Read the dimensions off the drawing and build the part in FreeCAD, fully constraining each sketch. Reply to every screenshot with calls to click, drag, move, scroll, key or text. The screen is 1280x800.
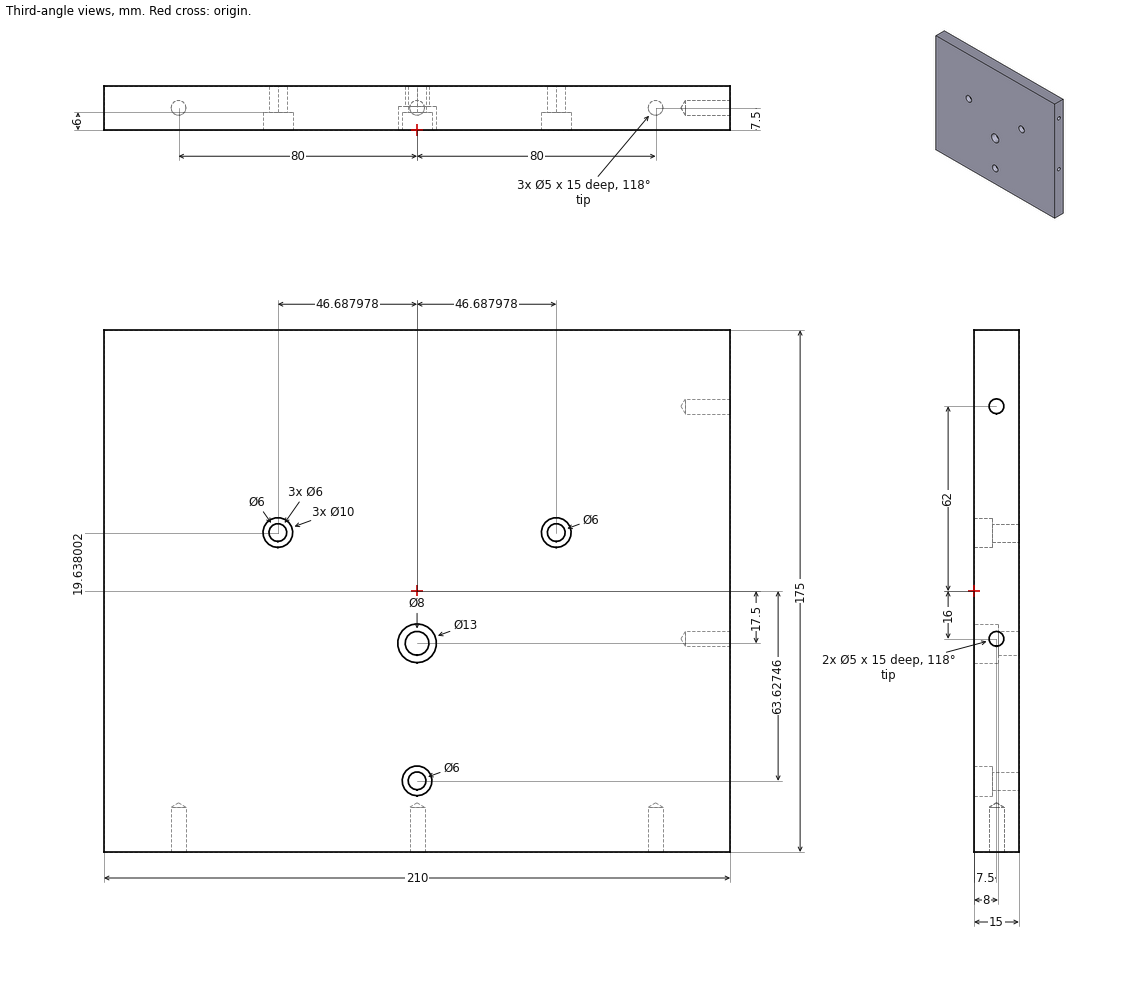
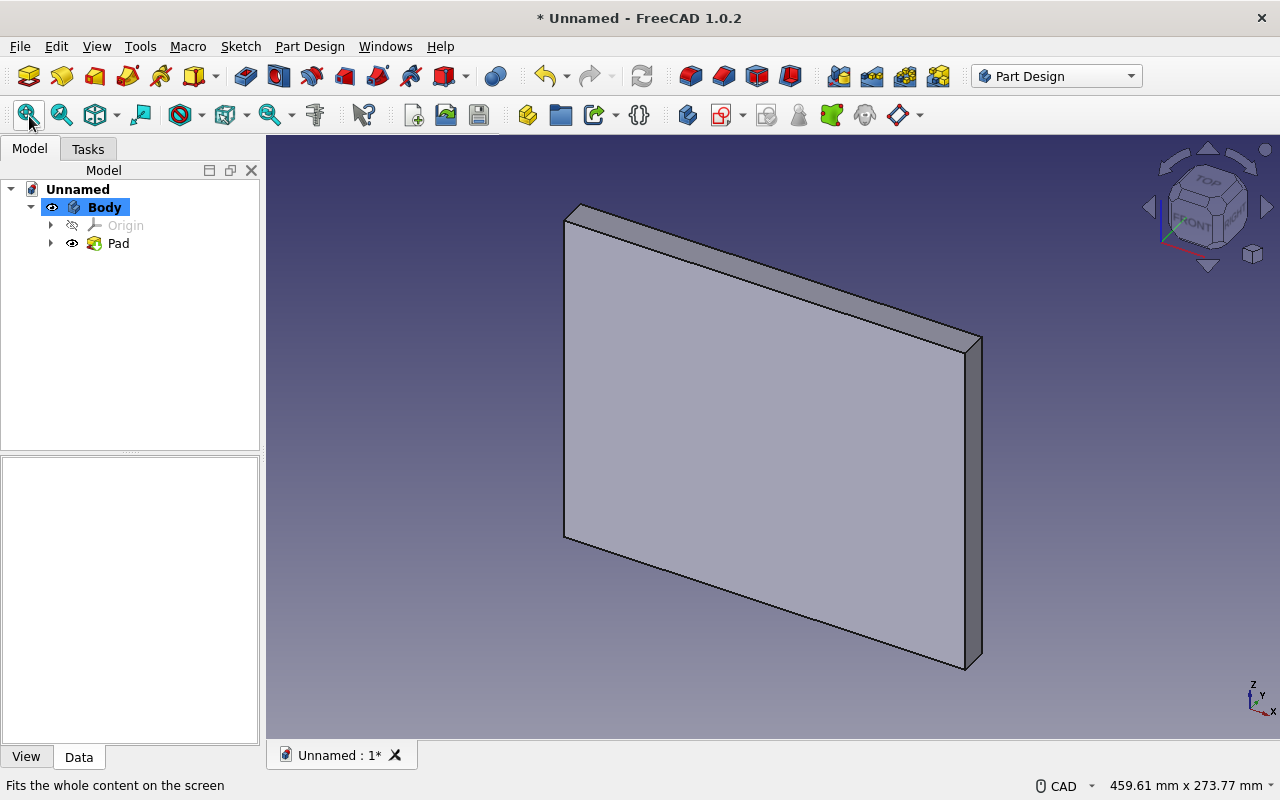
click(720, 116)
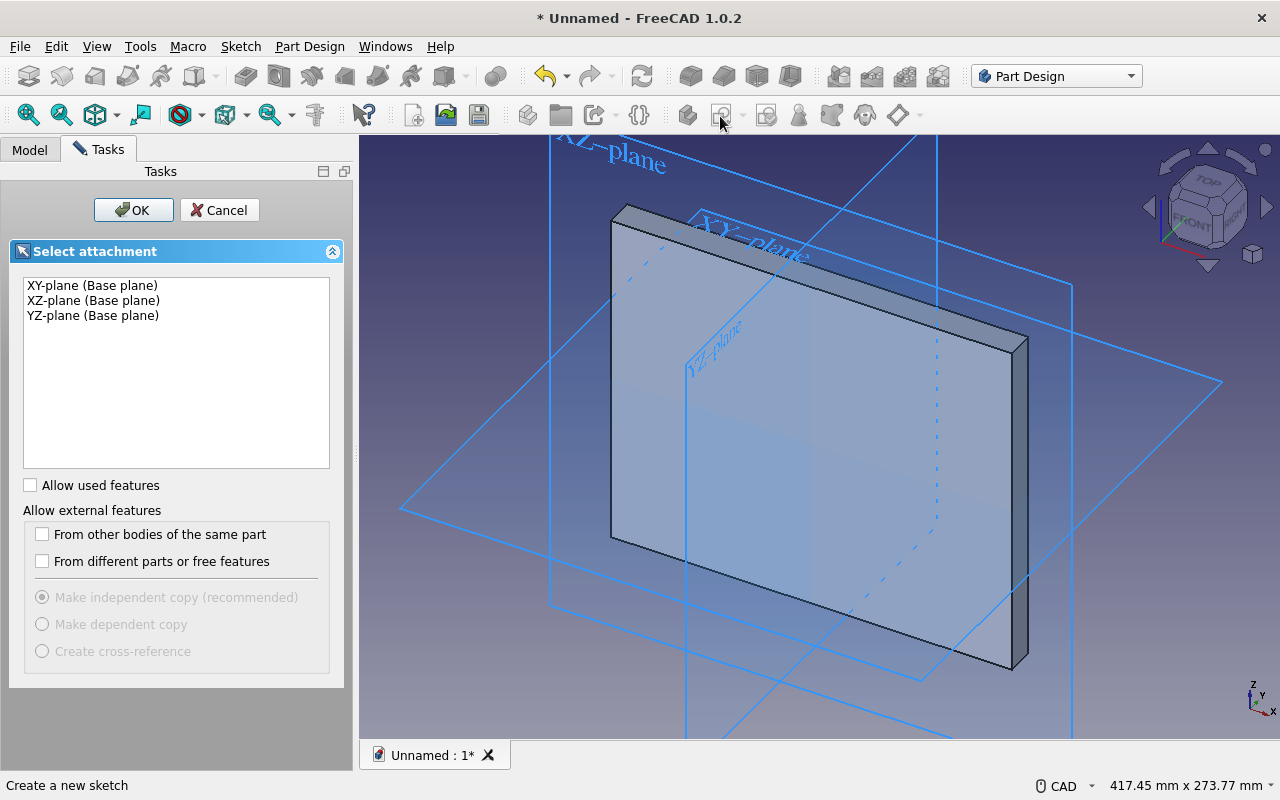
click(84, 300)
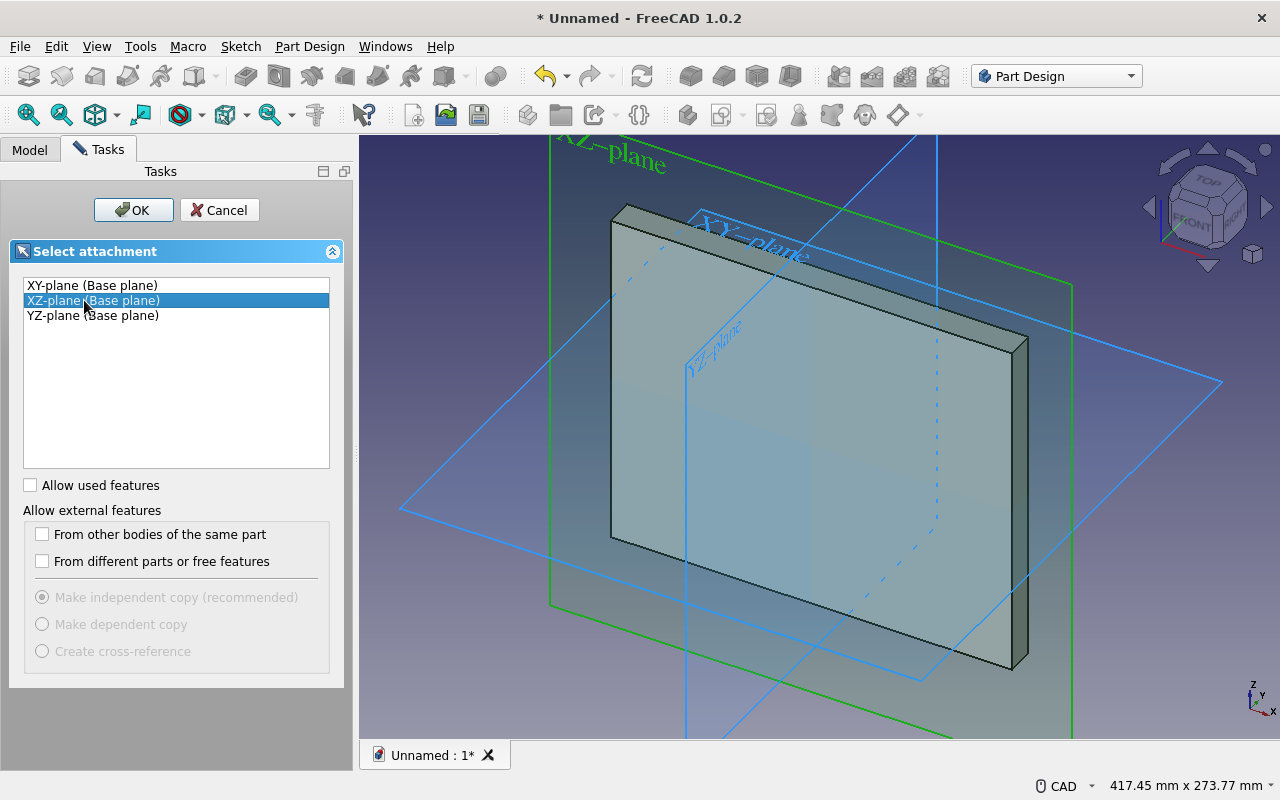
click(134, 210)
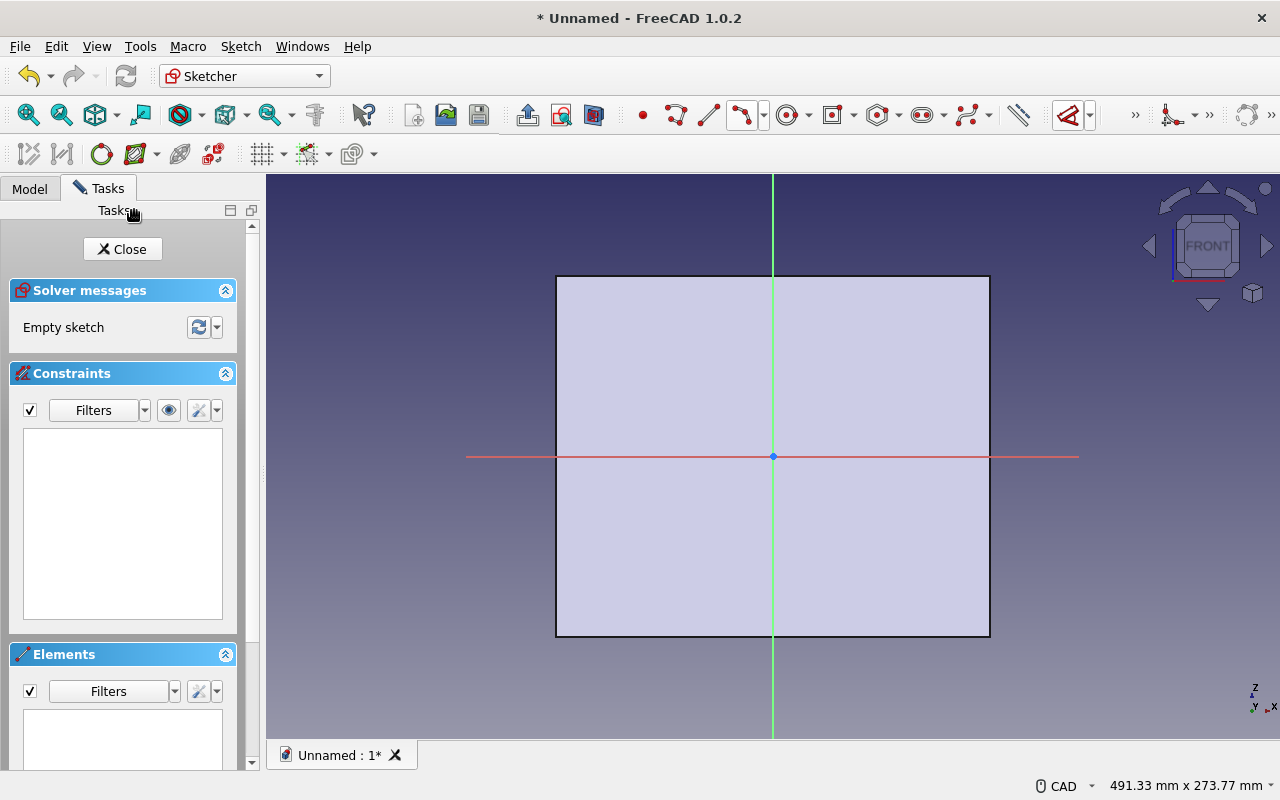
scroll(856, 557, up, 3)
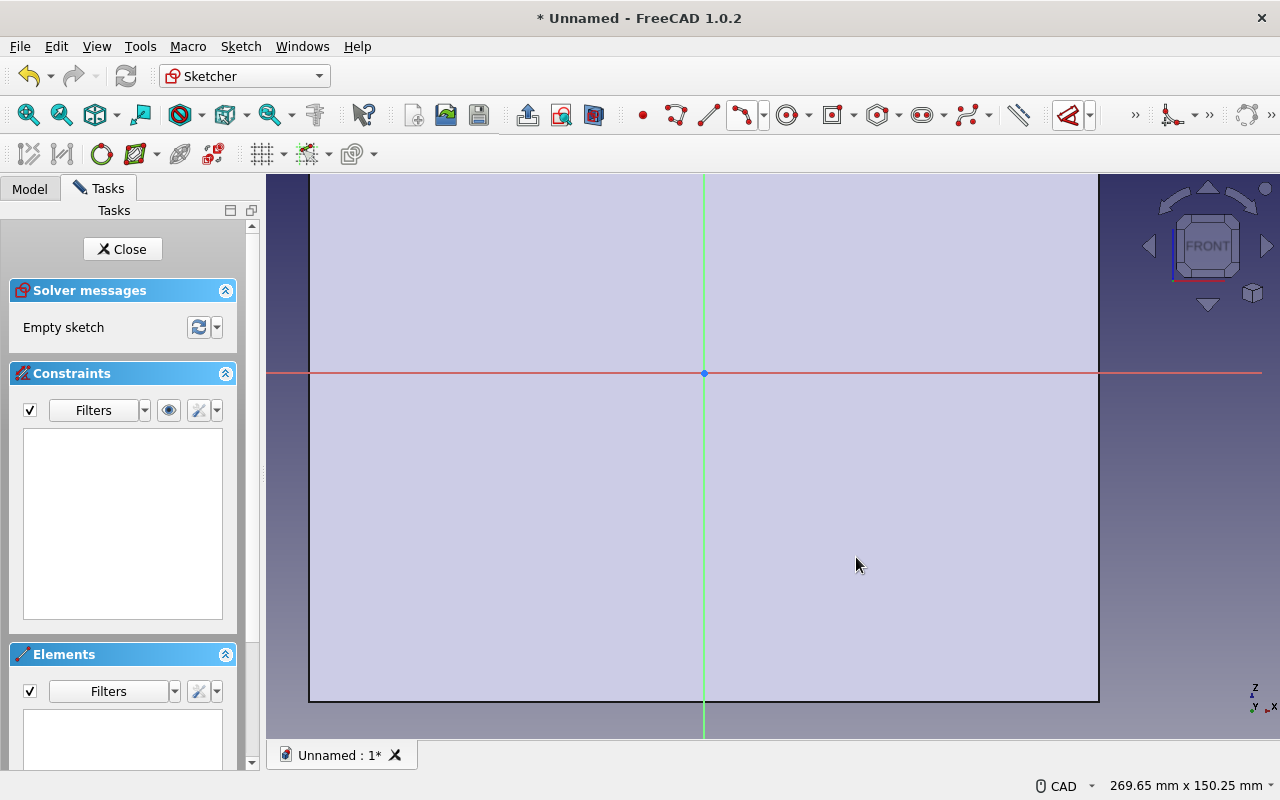
click(786, 116)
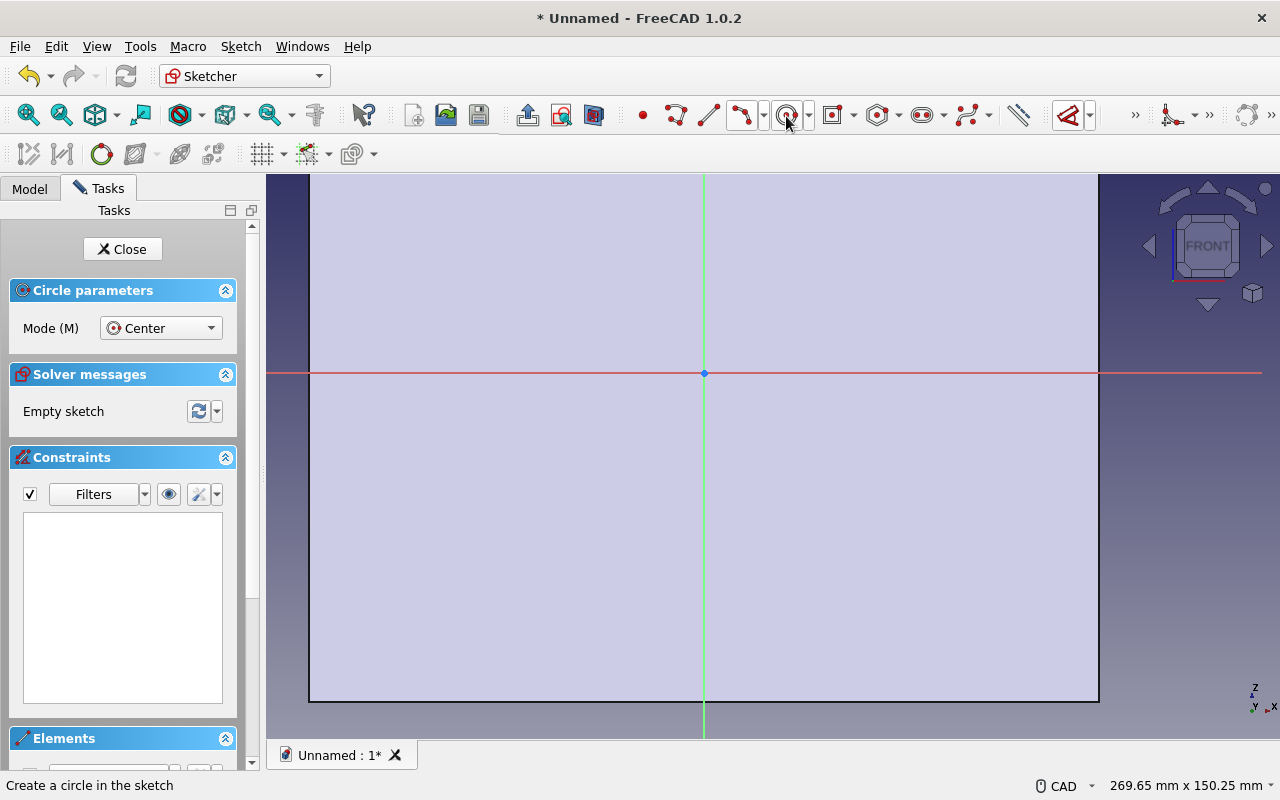
click(529, 299)
click(542, 286)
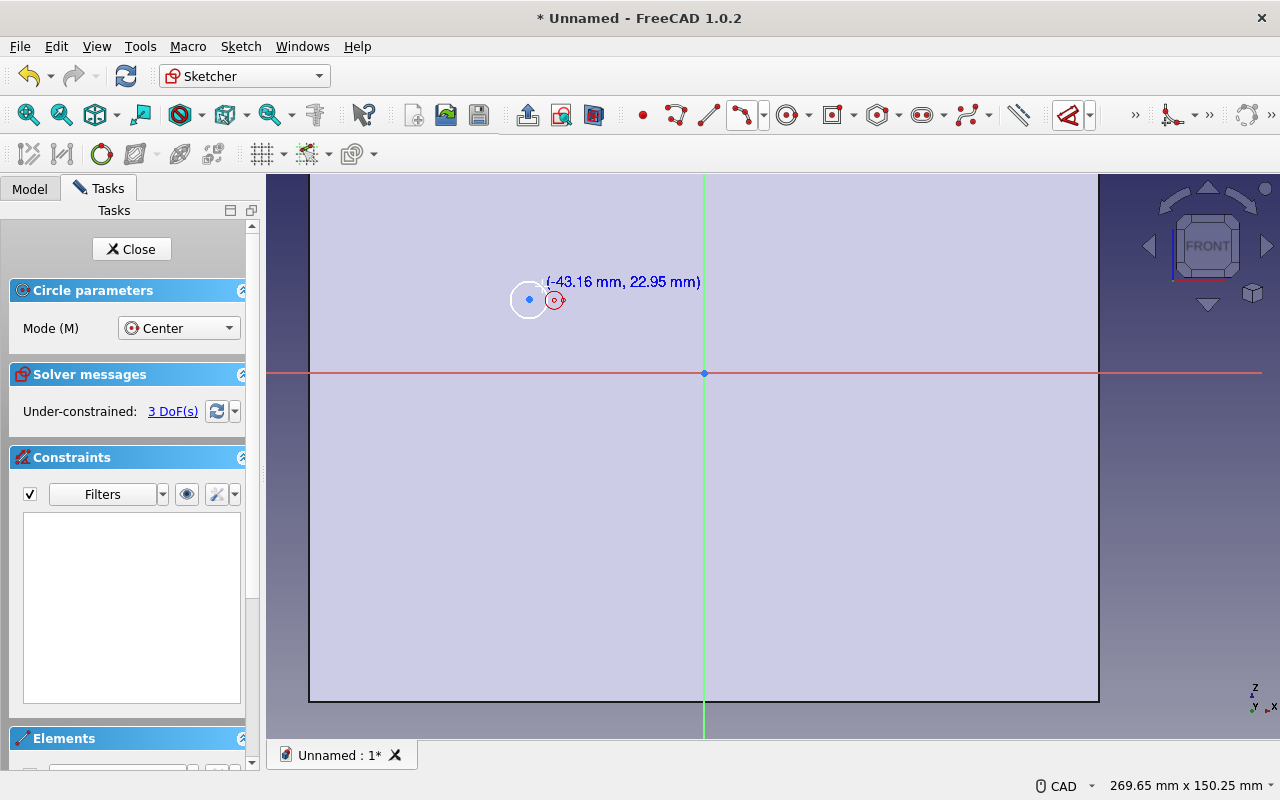
click(880, 299)
click(893, 286)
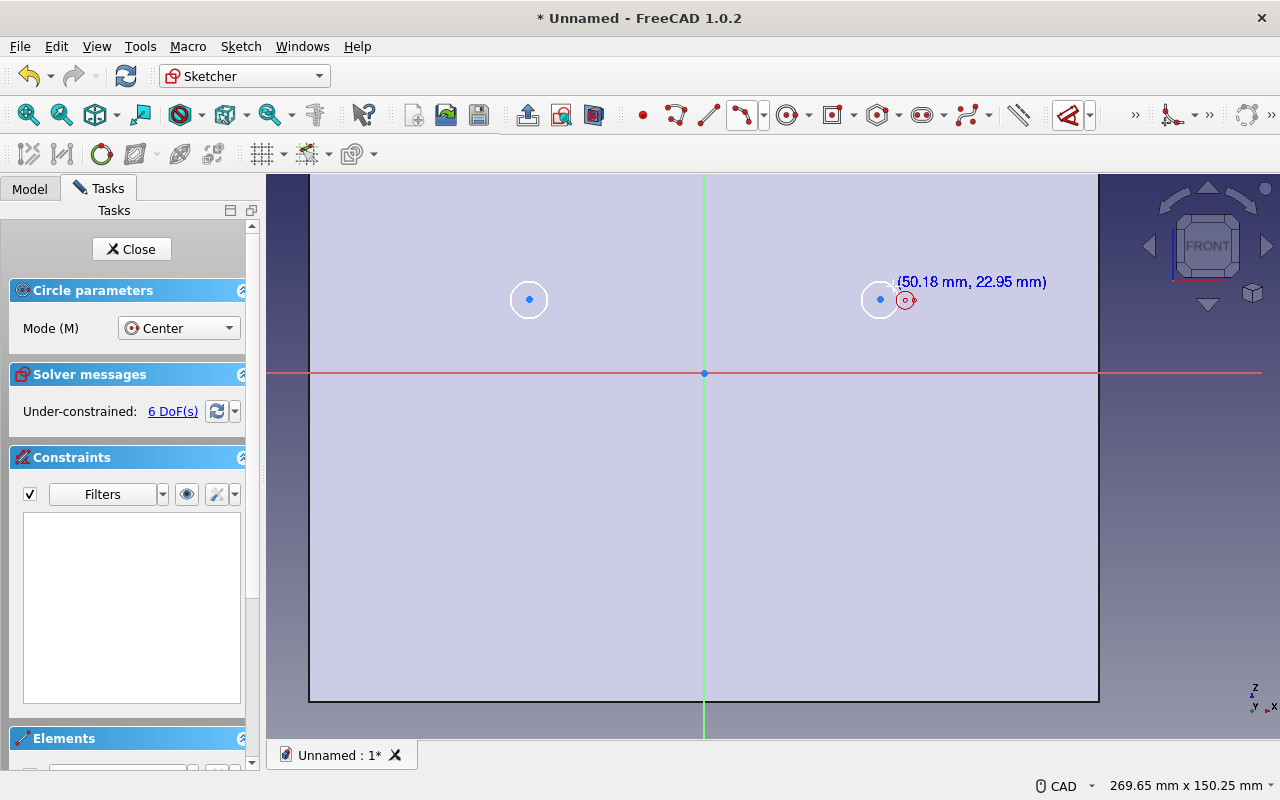
click(704, 613)
click(722, 606)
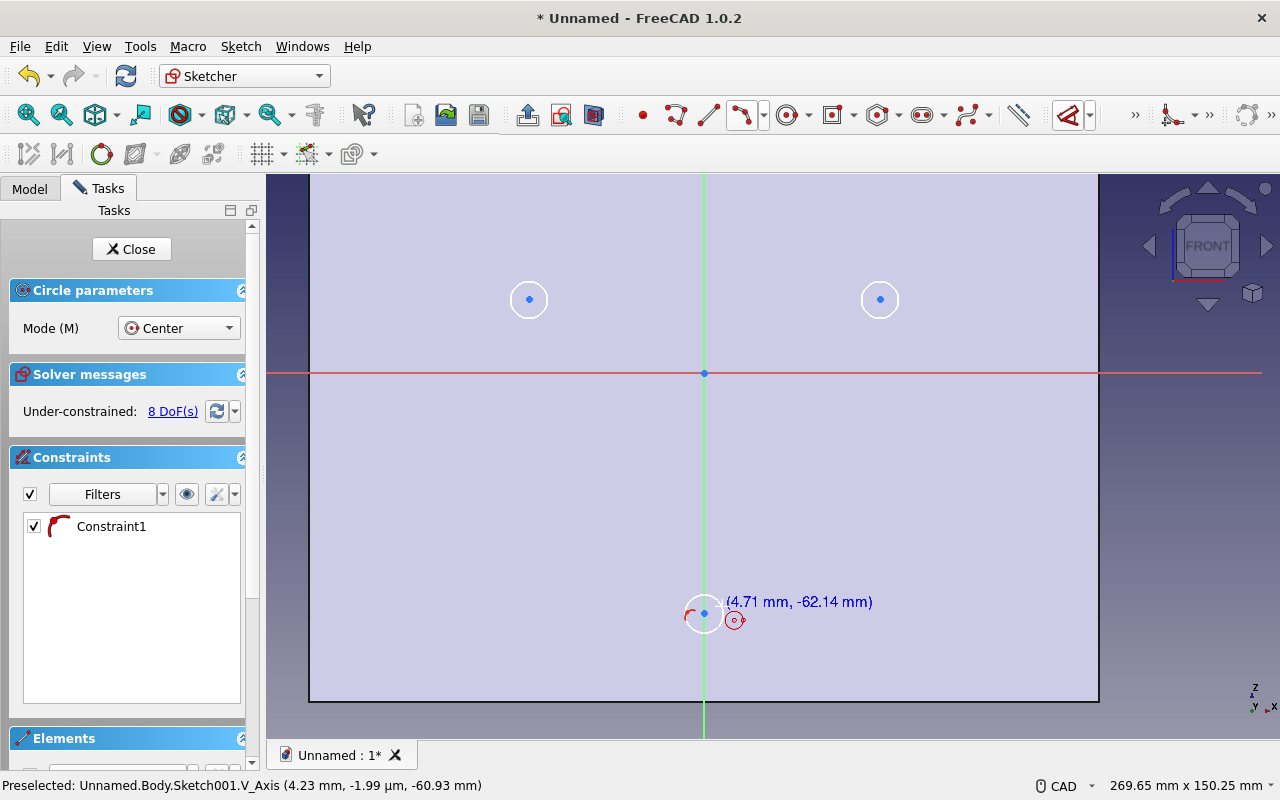
scroll(529, 299, up, 4)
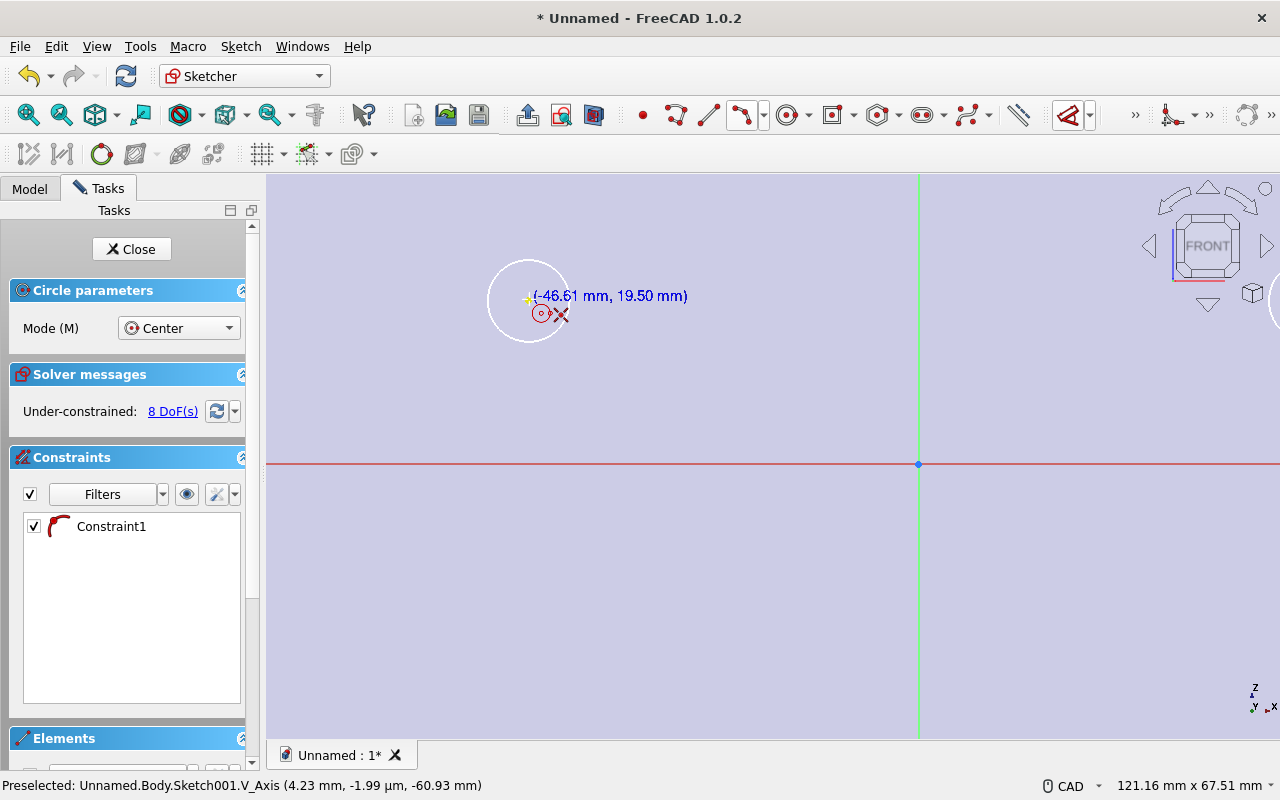
click(529, 301)
click(546, 282)